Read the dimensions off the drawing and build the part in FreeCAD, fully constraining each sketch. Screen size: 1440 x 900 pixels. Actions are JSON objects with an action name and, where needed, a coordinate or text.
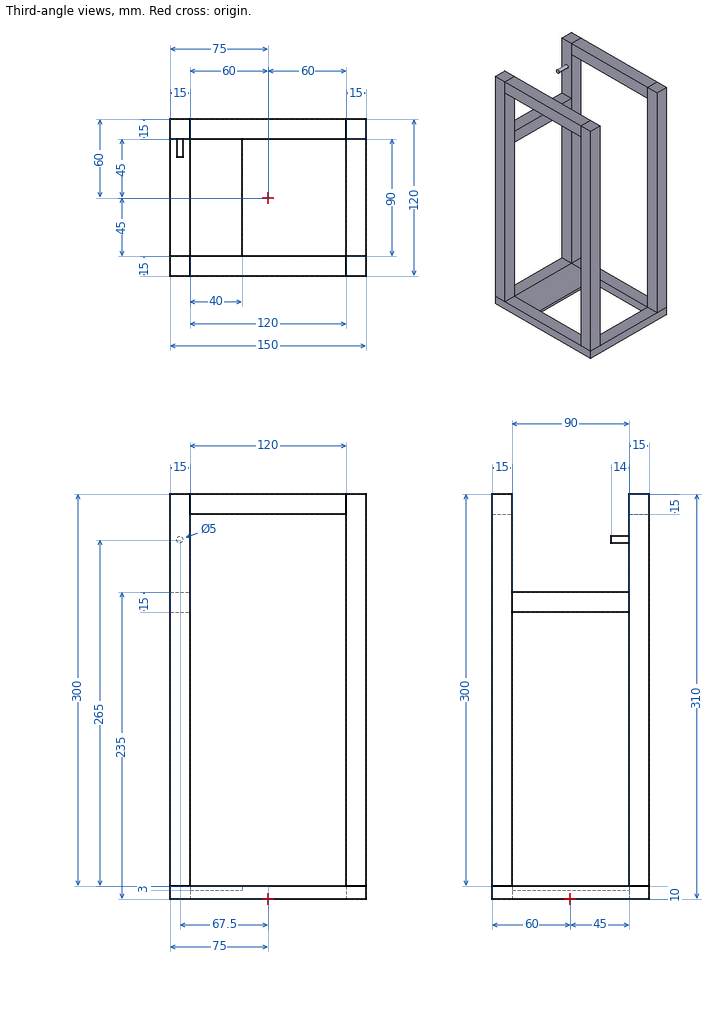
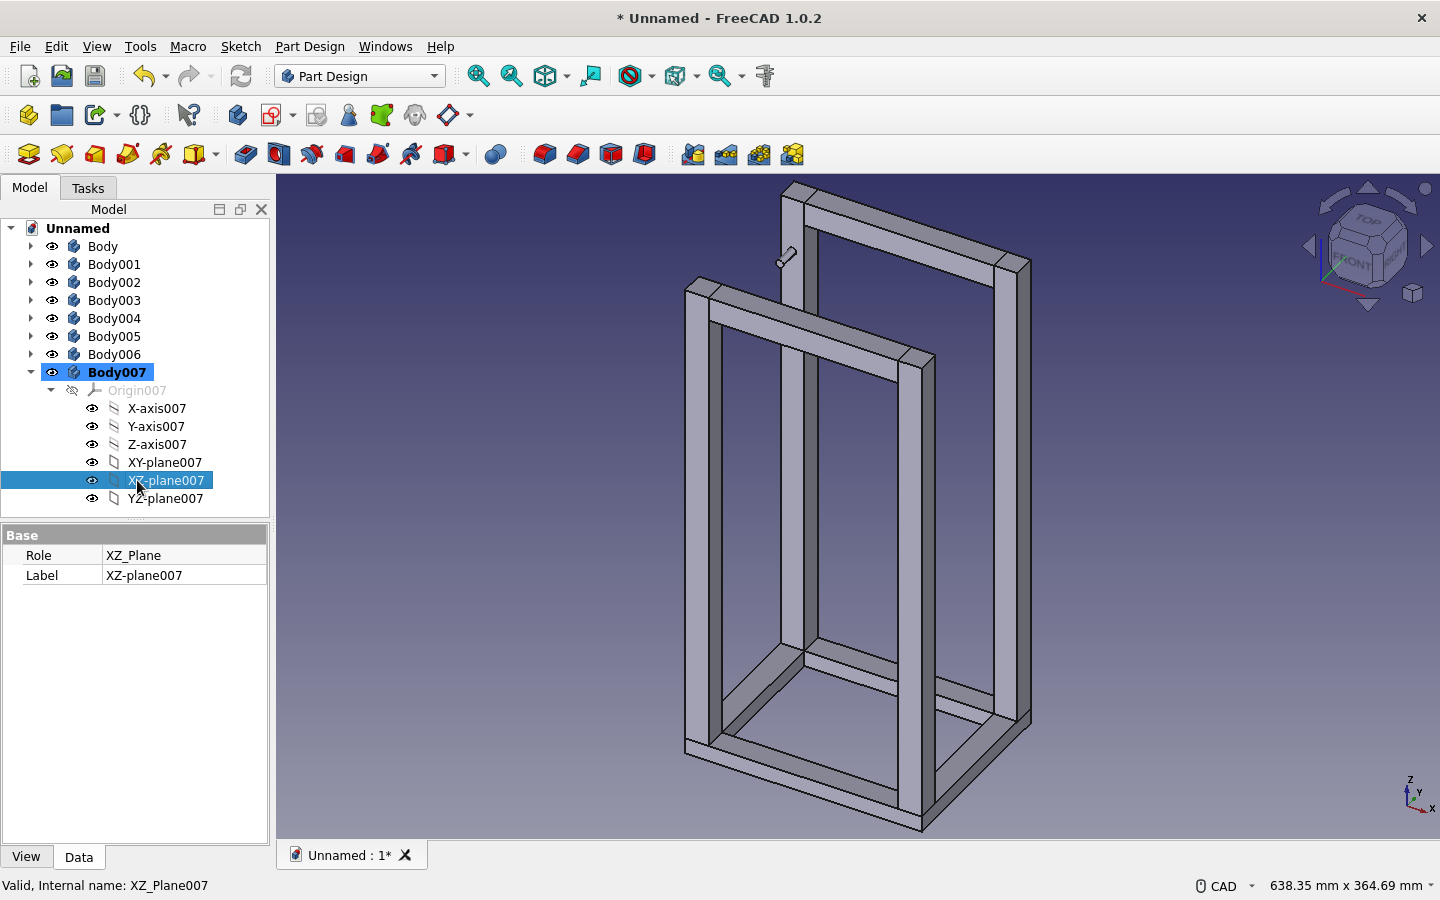
{"action": "left_click", "coordinate": [448, 116]}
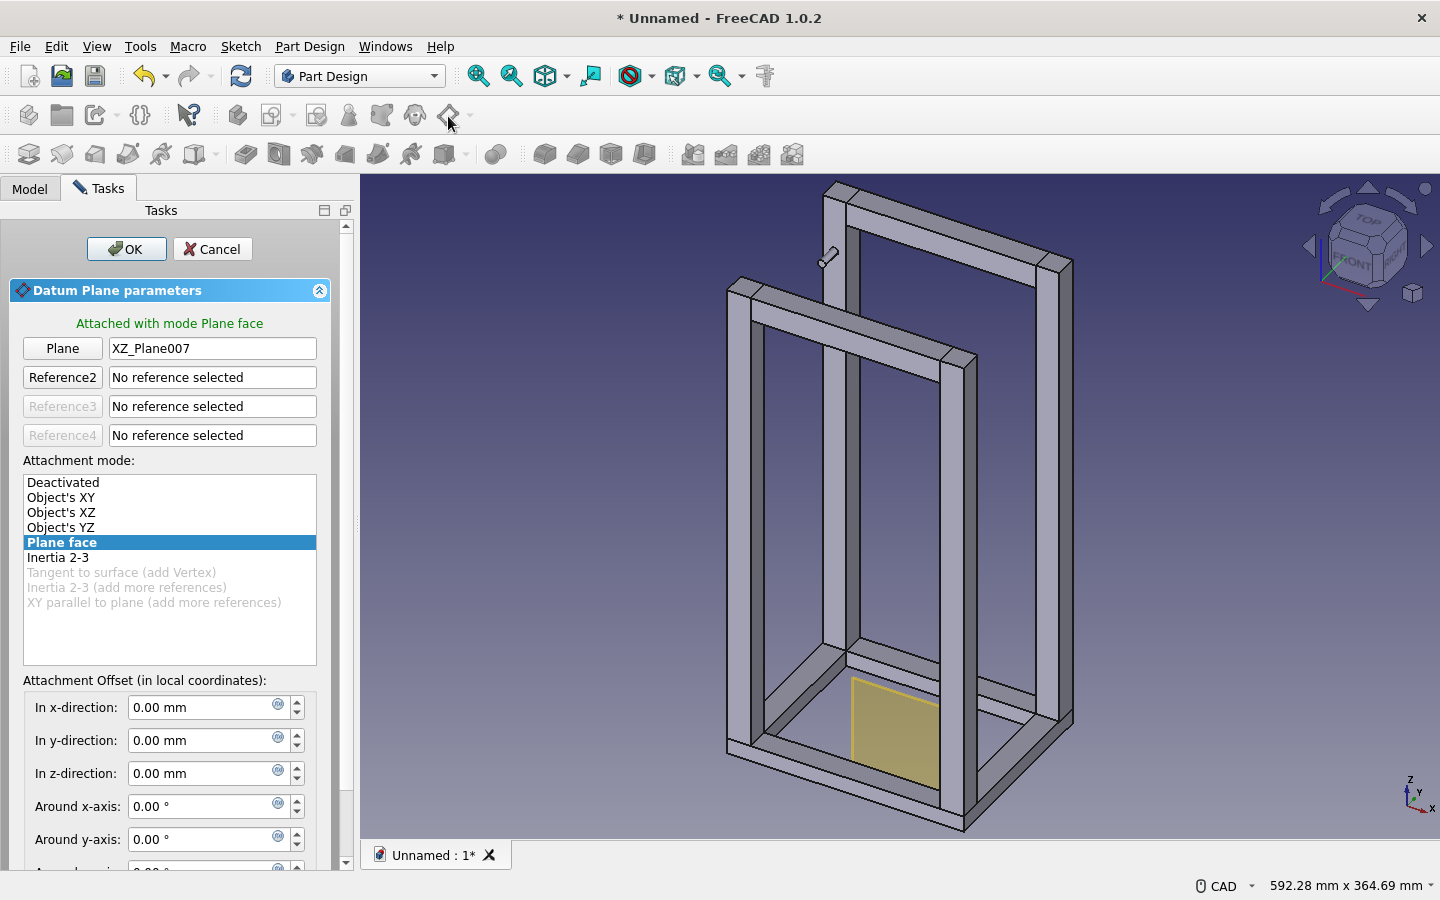
{"action": "triple_click", "coordinate": [210, 774]}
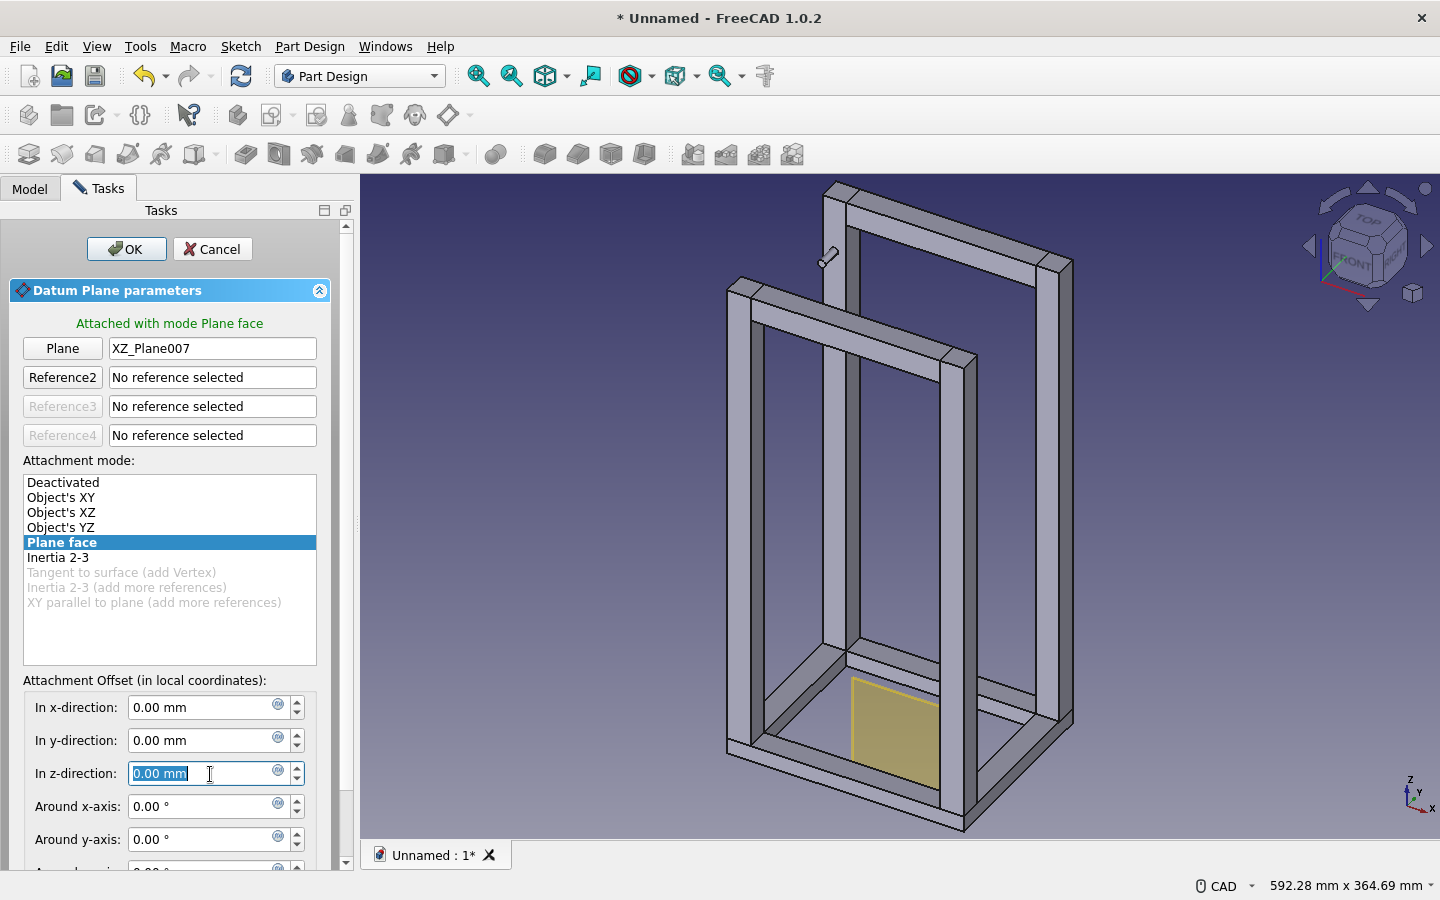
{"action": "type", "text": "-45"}
{"action": "key", "text": "Tab"}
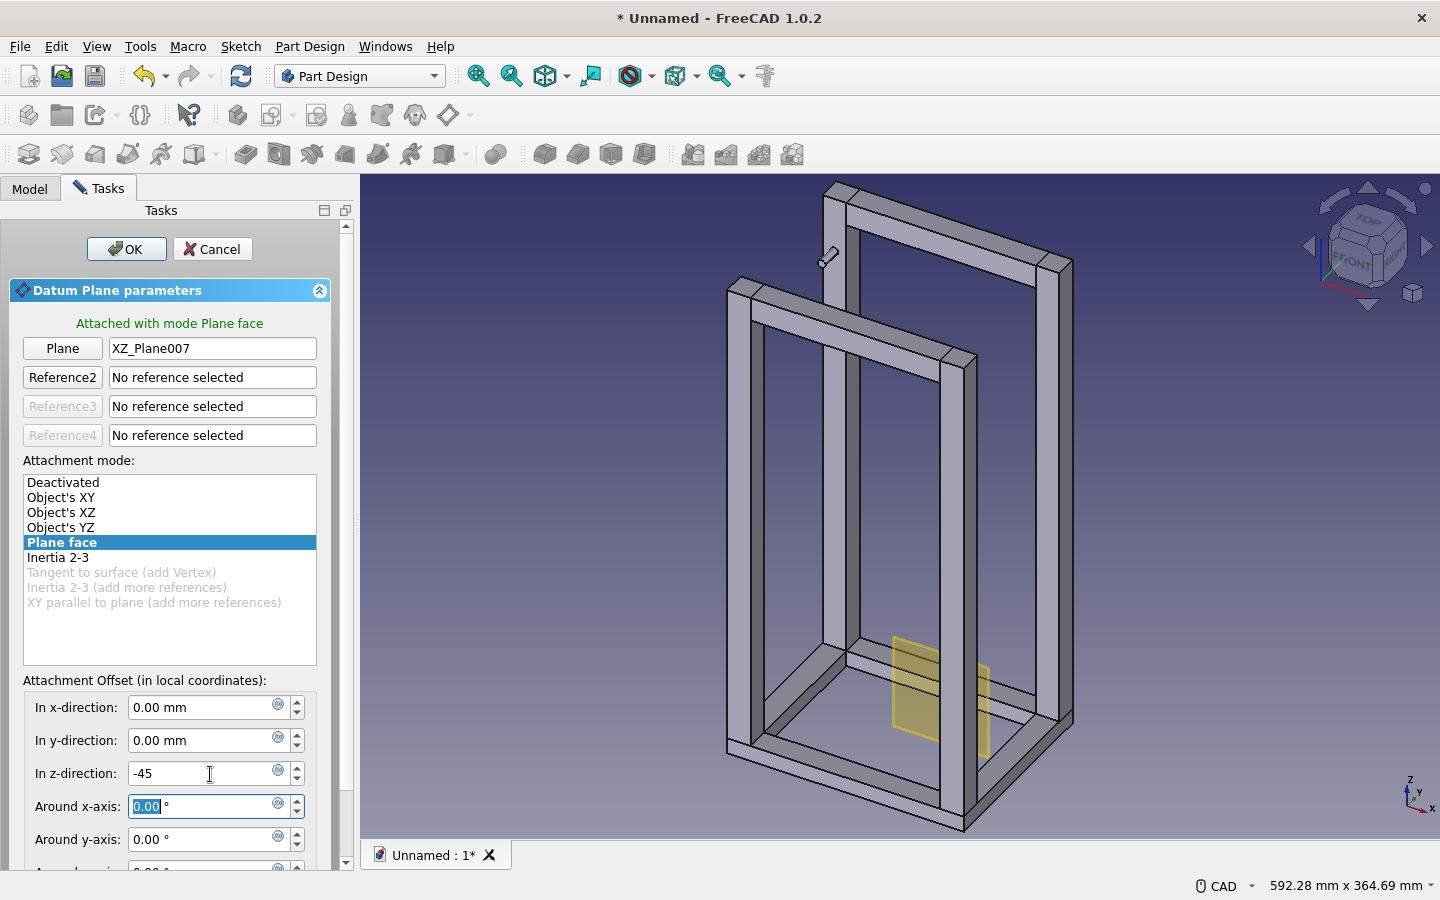
{"action": "left_click", "coordinate": [127, 249]}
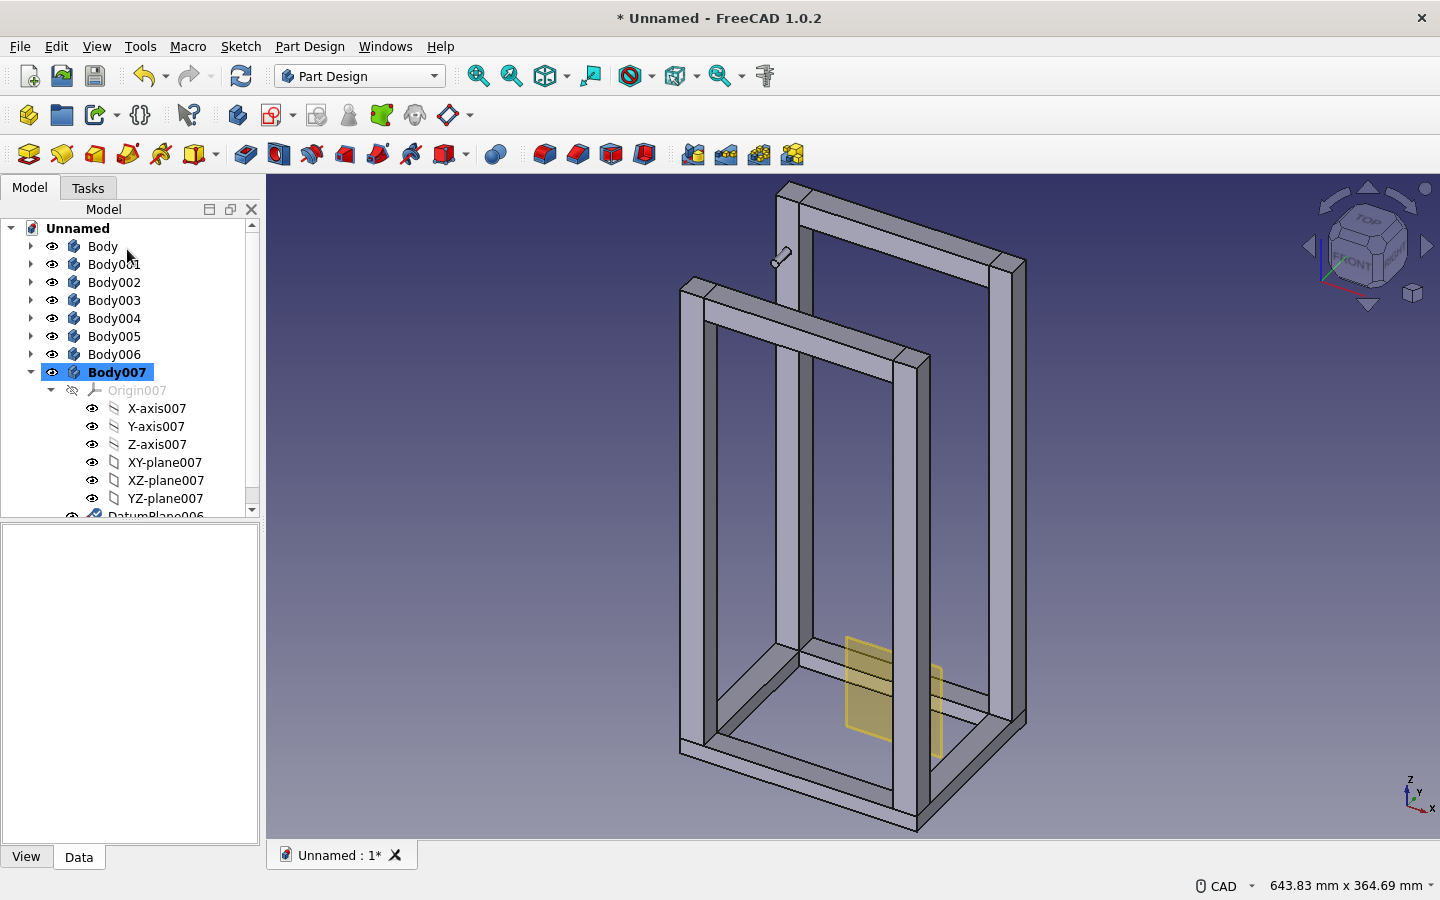
{"action": "left_click", "coordinate": [117, 516]}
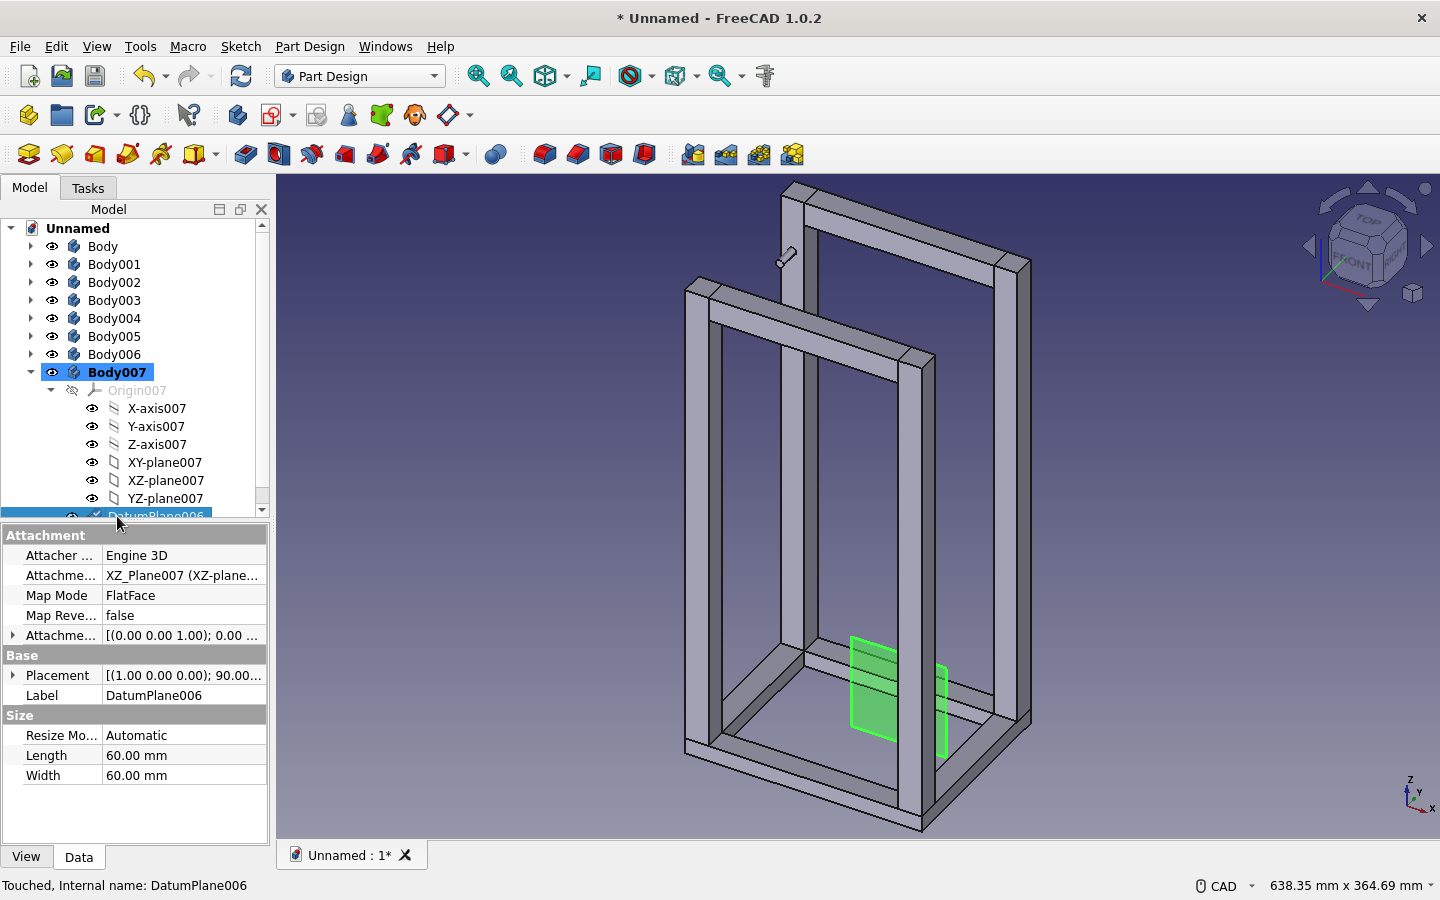
{"action": "left_click", "coordinate": [270, 116]}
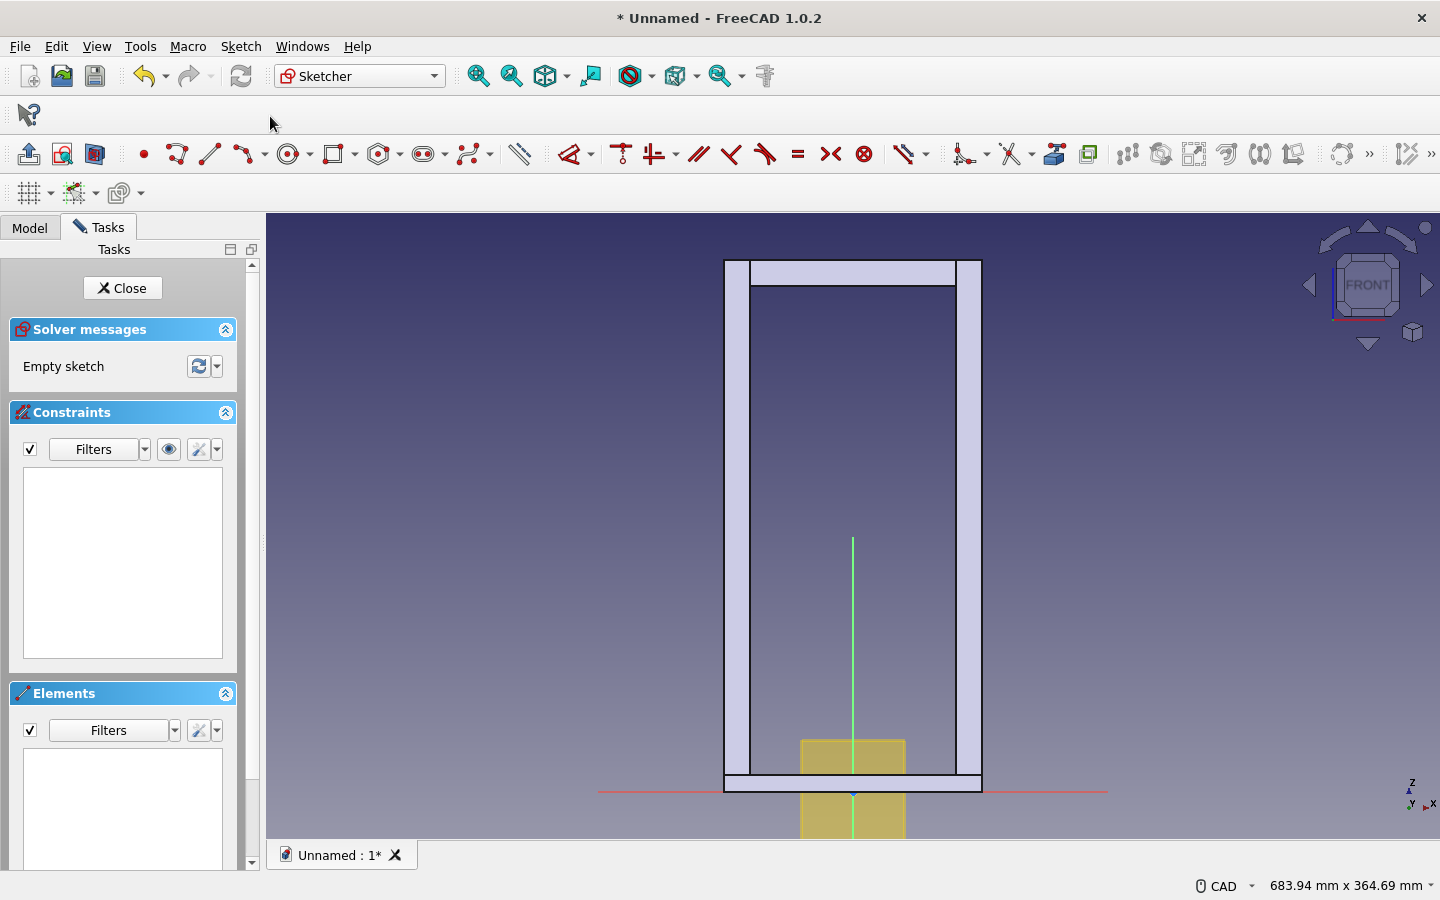
{"action": "scroll", "coordinate": [734, 393], "scroll_direction": "up", "scroll_amount": 14}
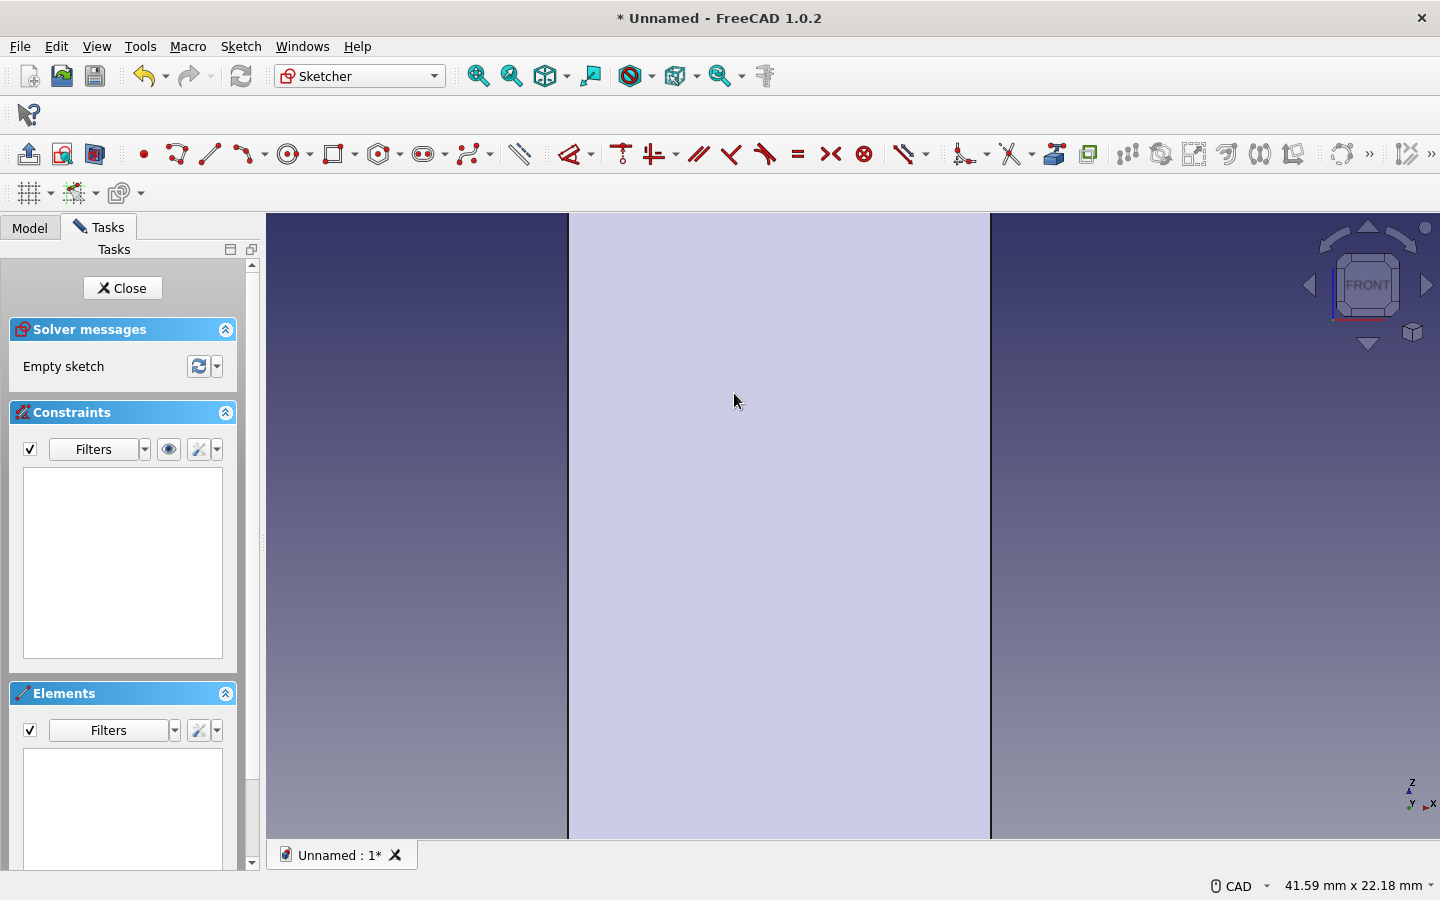
{"action": "left_click", "coordinate": [332, 154]}